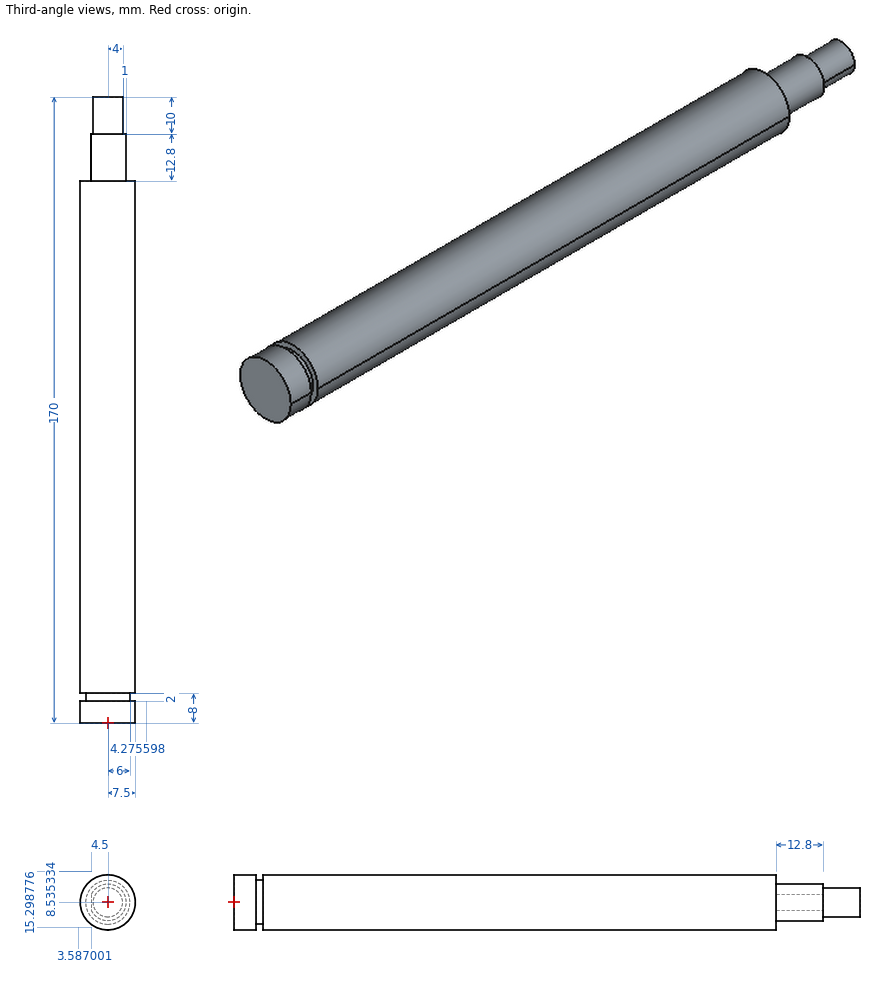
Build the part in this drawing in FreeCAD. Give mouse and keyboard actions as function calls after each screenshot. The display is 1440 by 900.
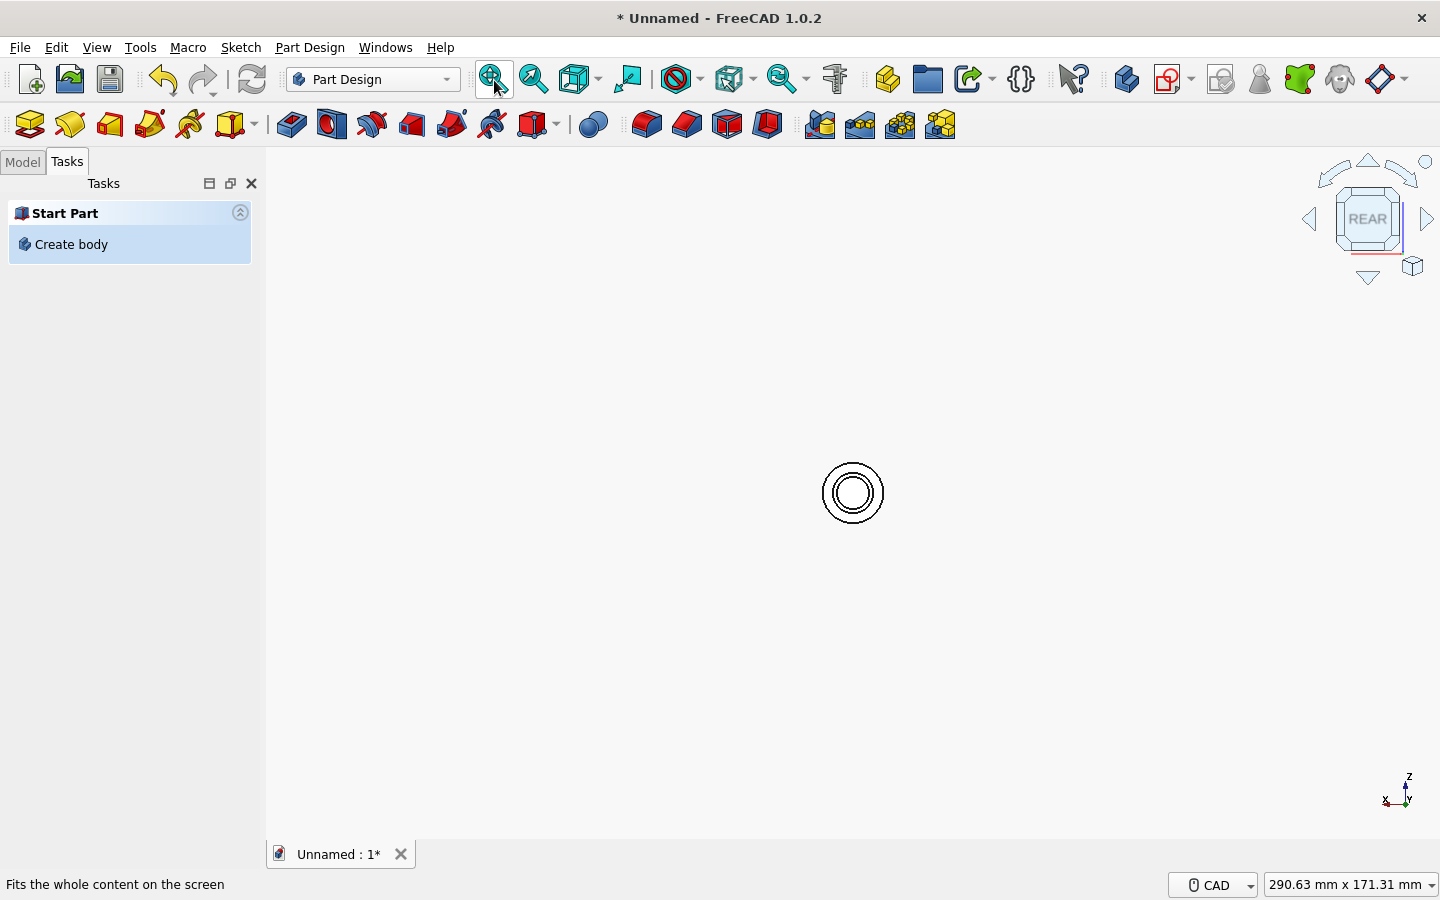
scroll(859, 509, up, 10)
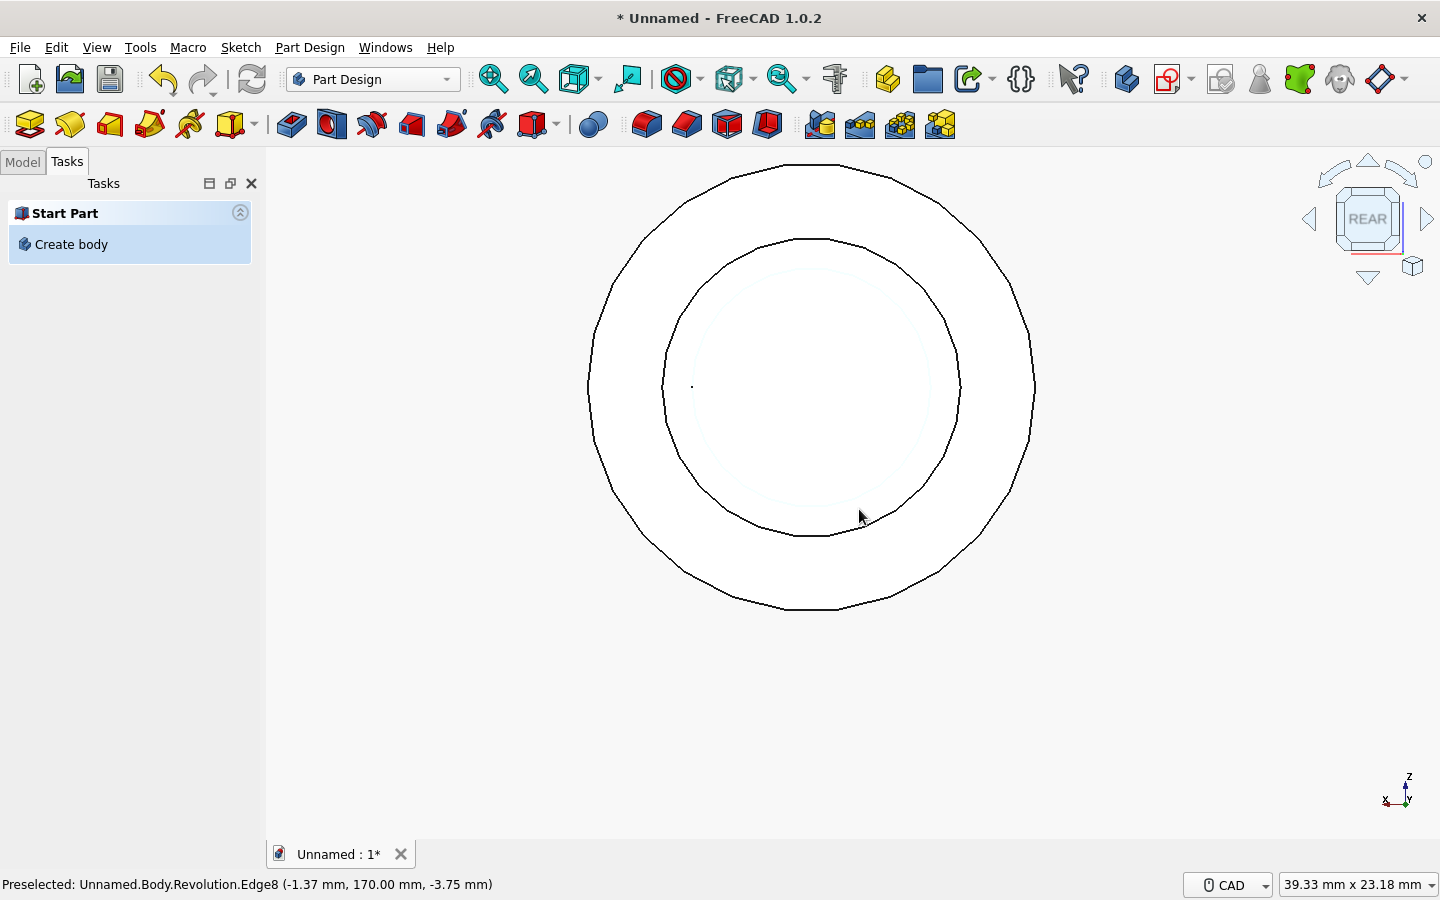
click(854, 514)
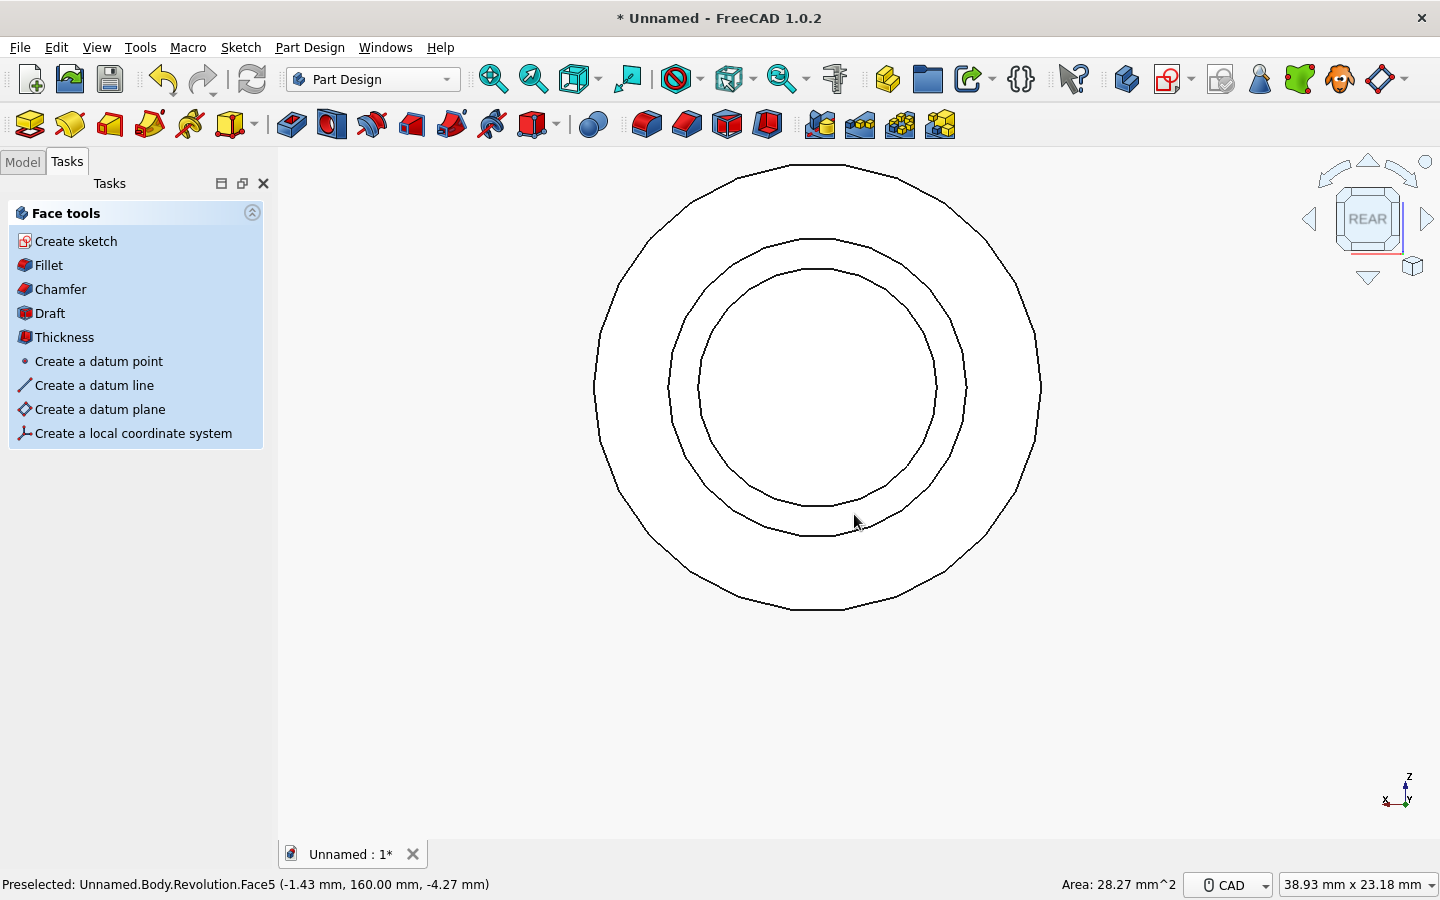
click(1168, 80)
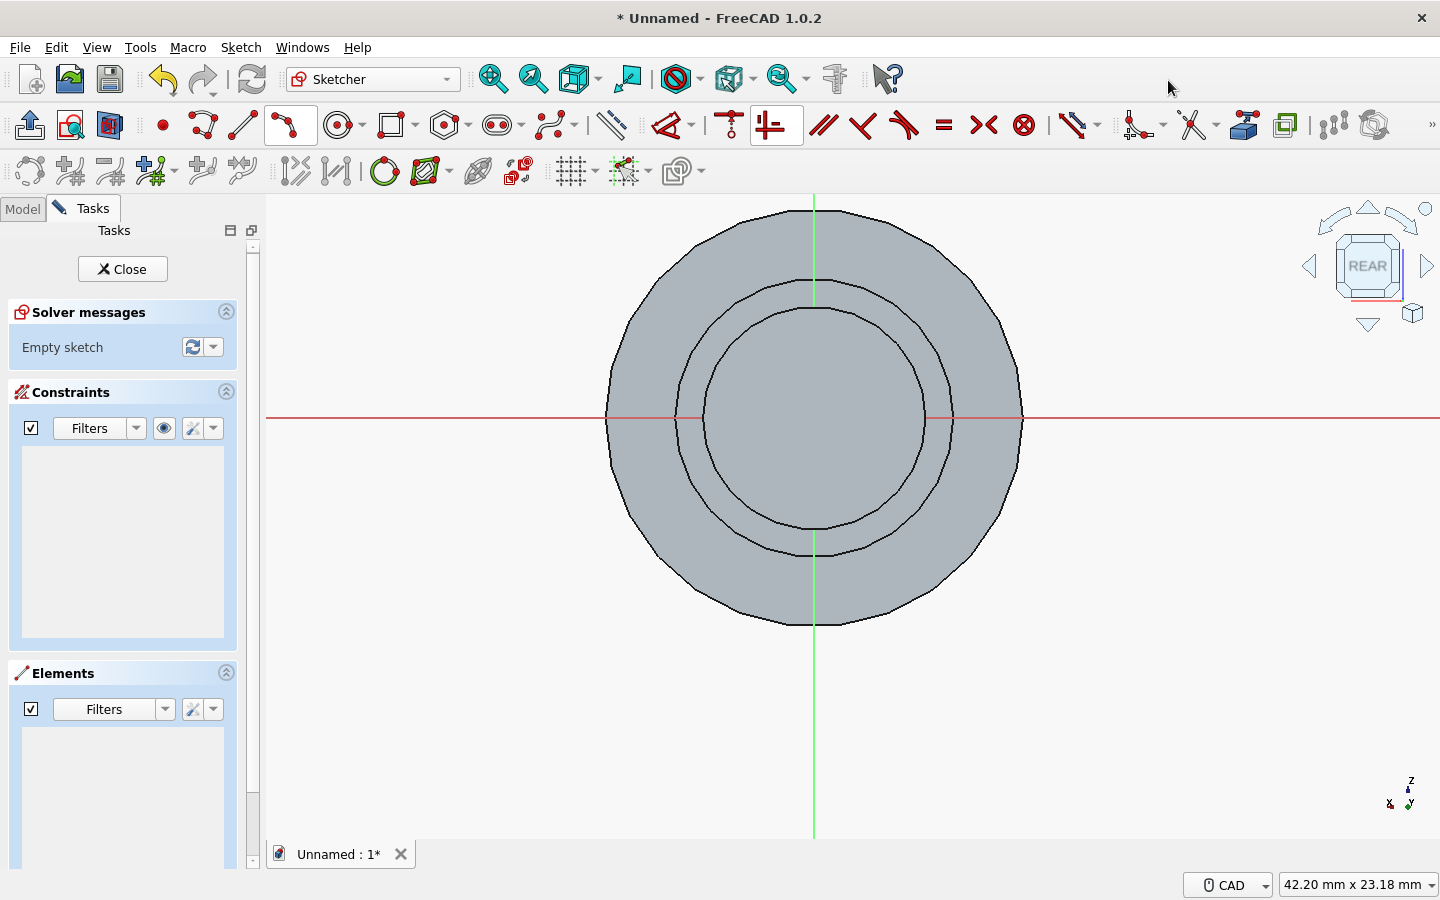
scroll(294, 811, down, 1)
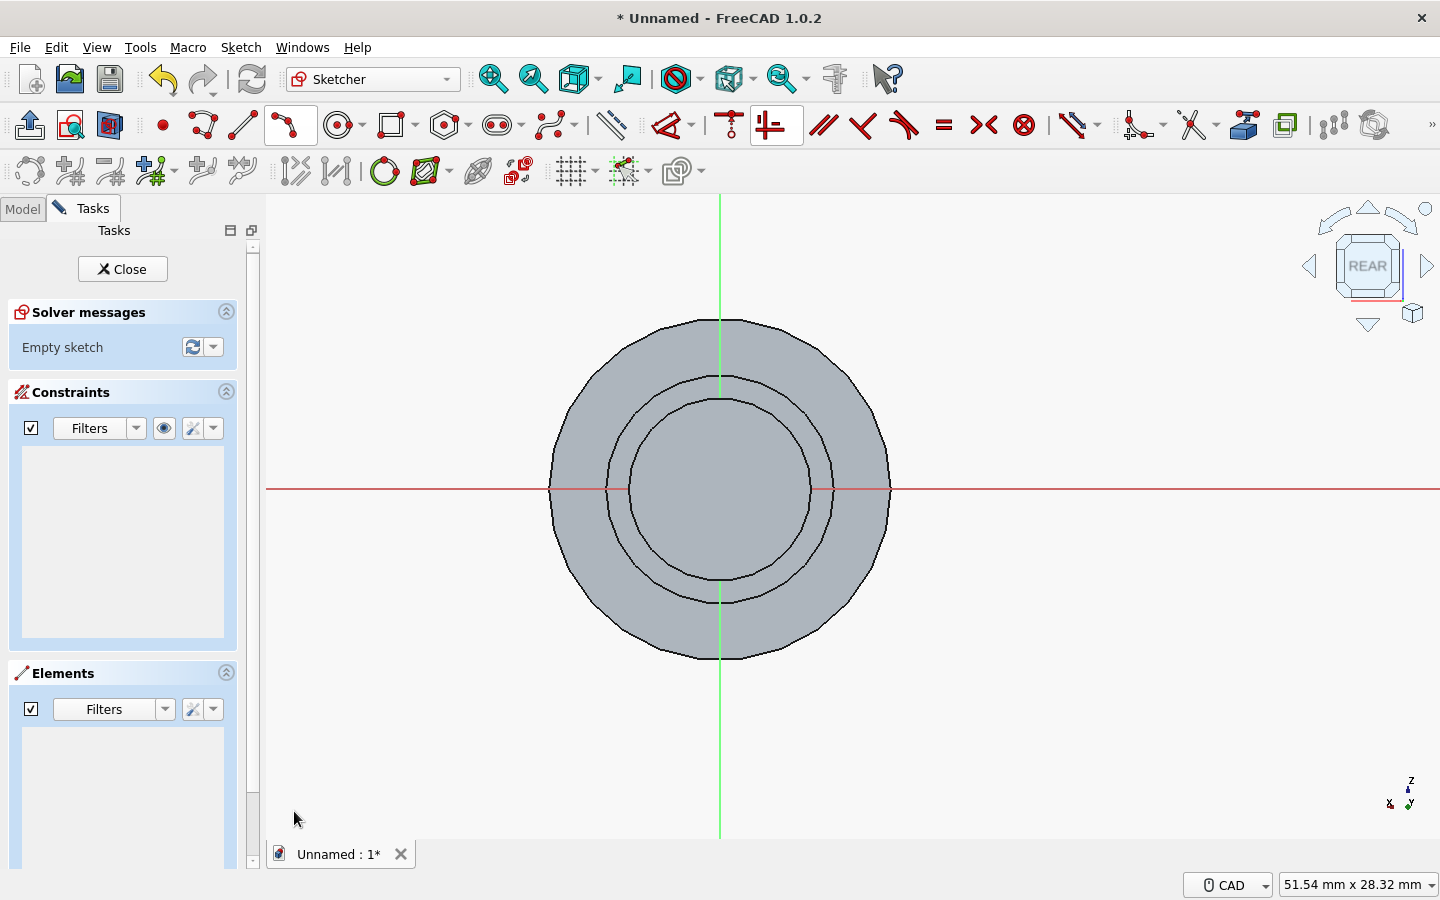
click(392, 126)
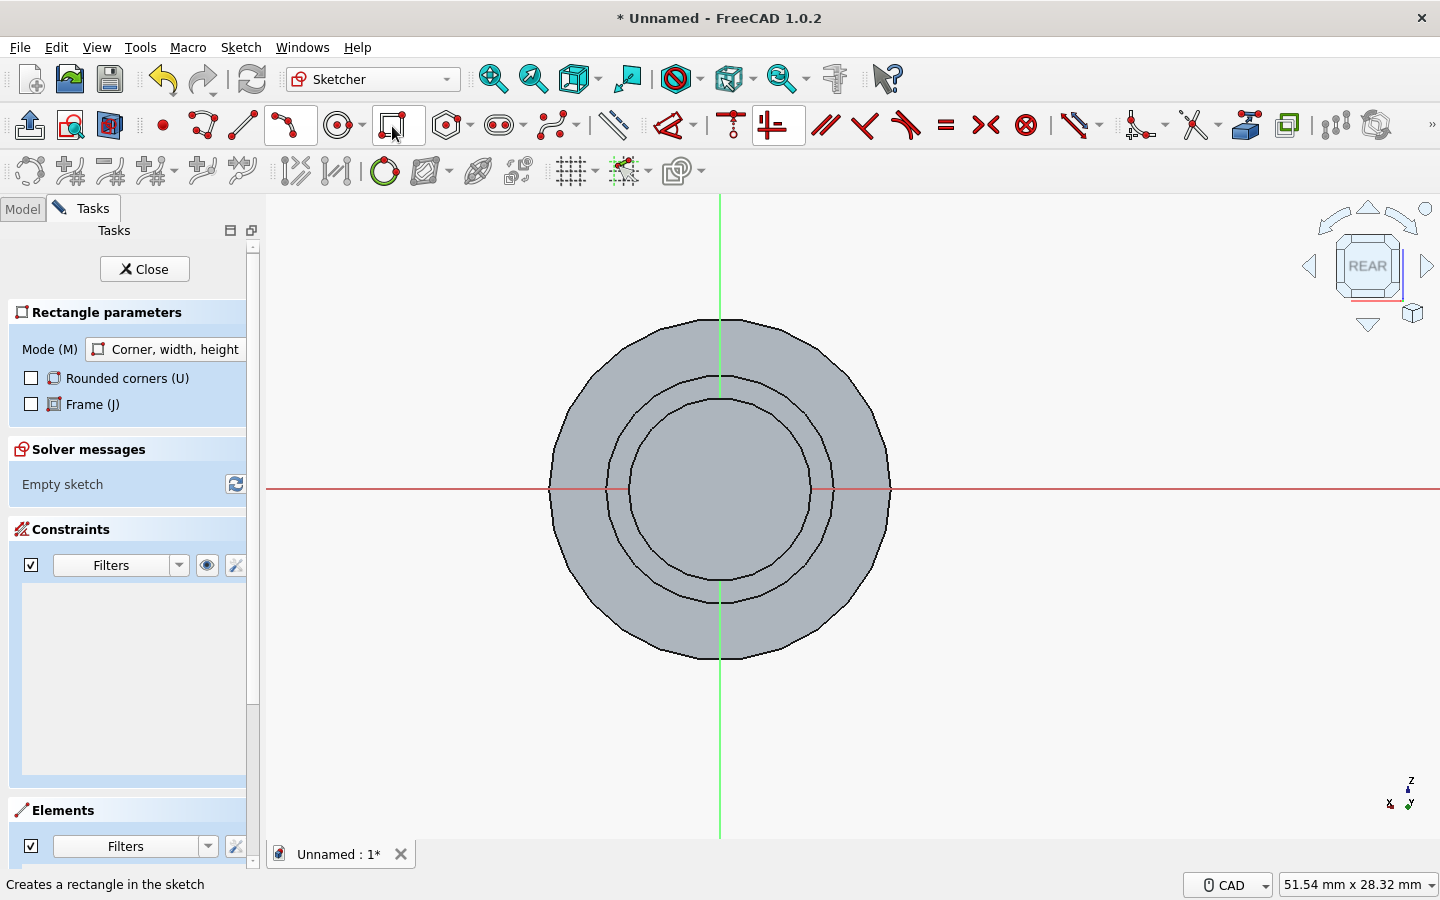
click(822, 295)
click(904, 644)
key(Escape)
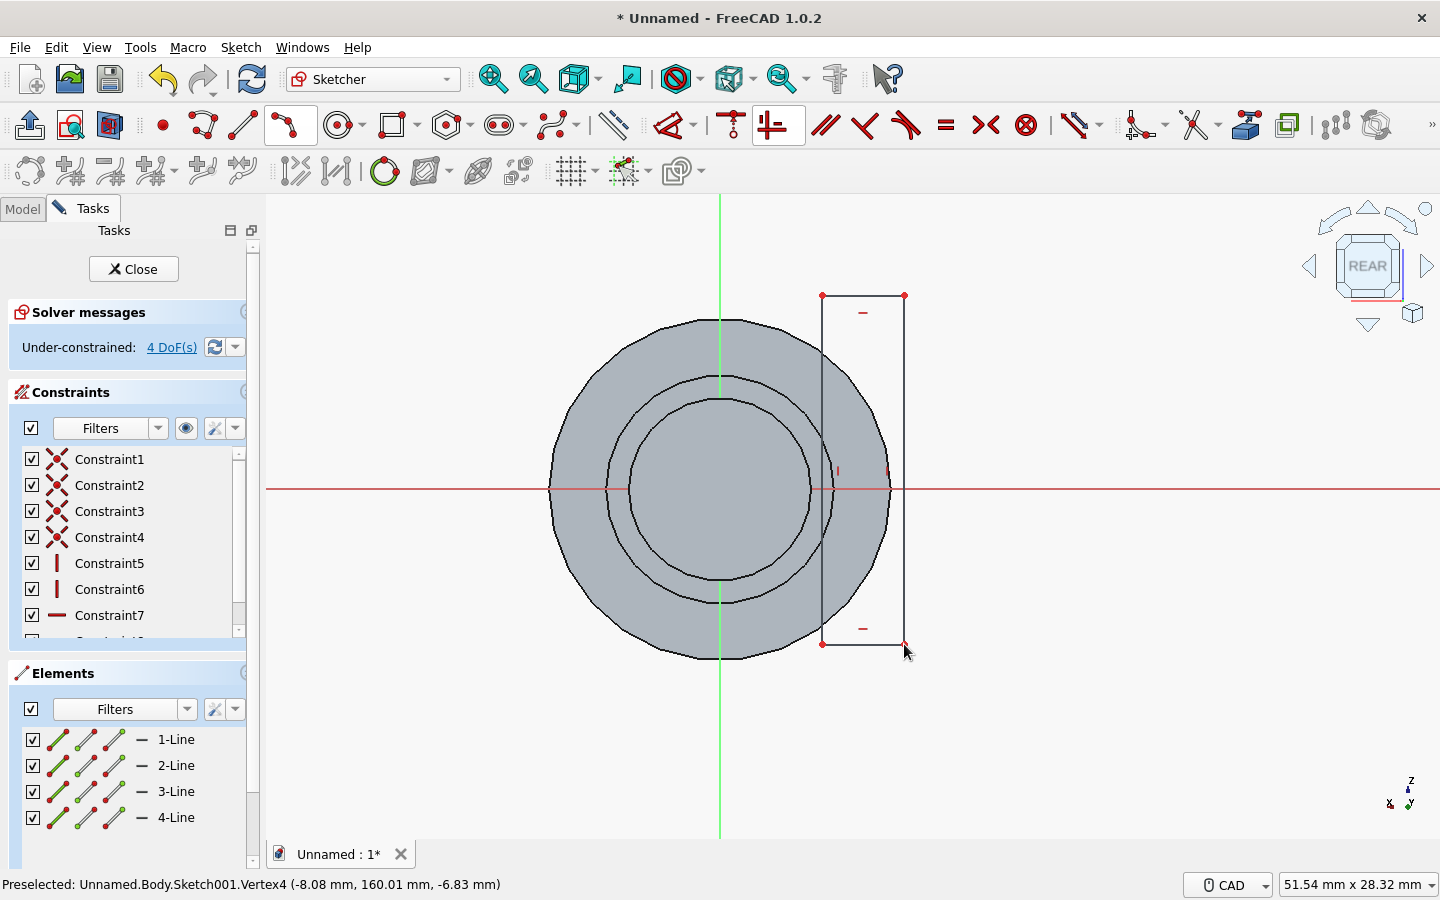
click(668, 126)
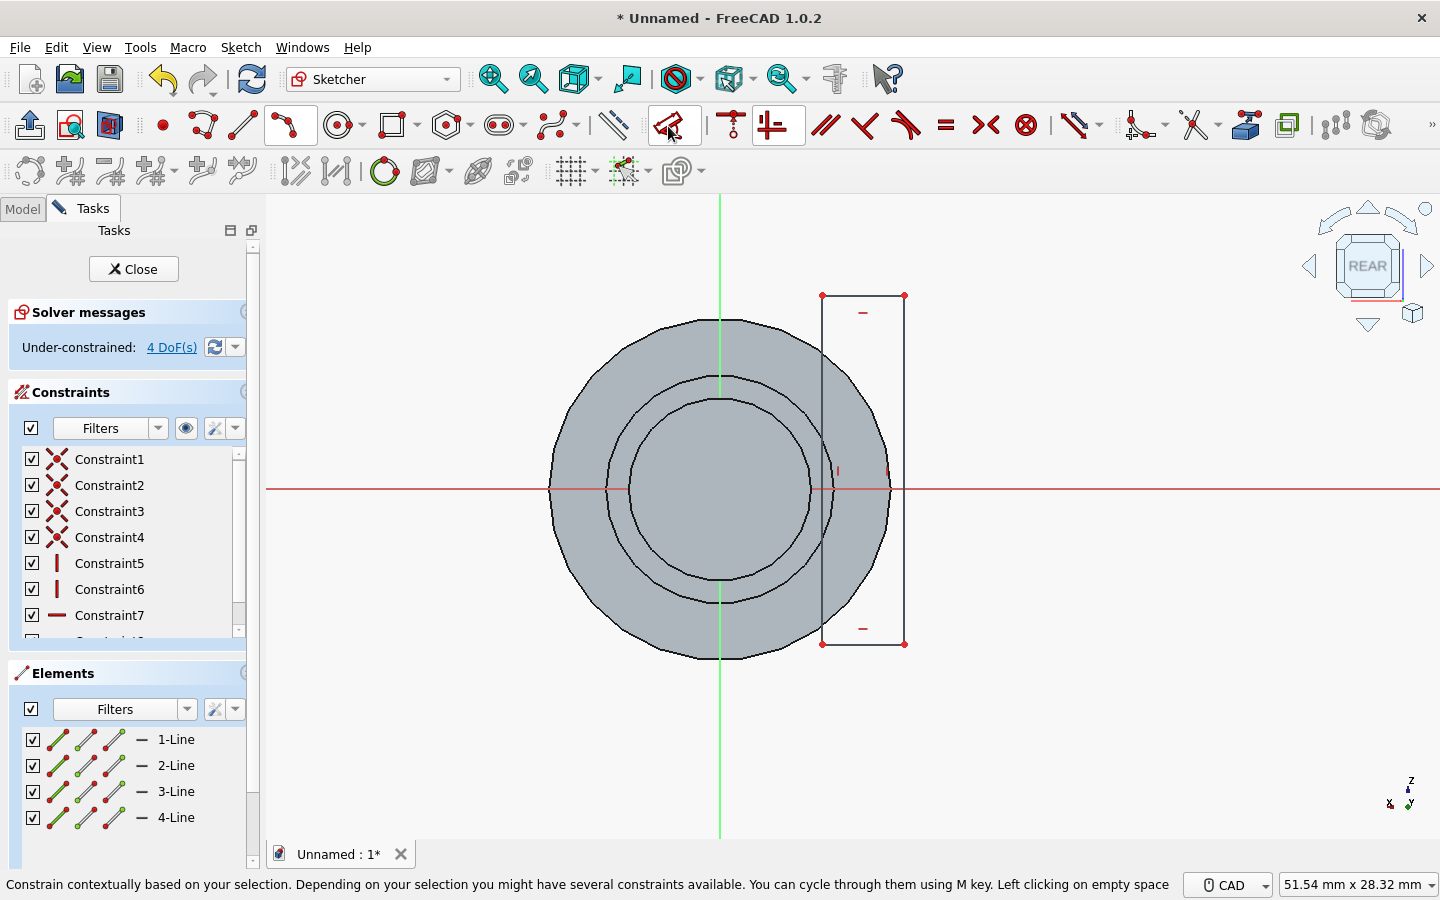
click(822, 296)
click(771, 262)